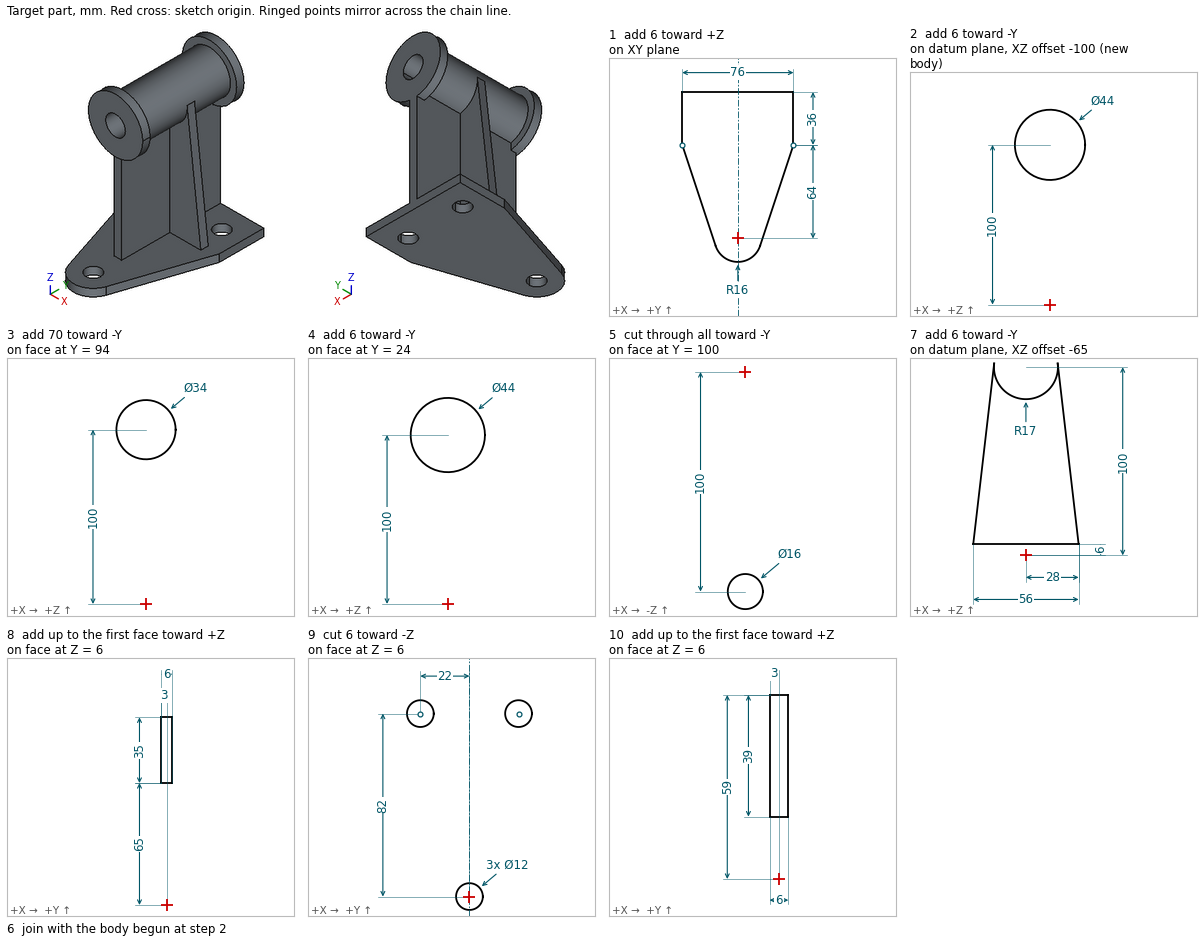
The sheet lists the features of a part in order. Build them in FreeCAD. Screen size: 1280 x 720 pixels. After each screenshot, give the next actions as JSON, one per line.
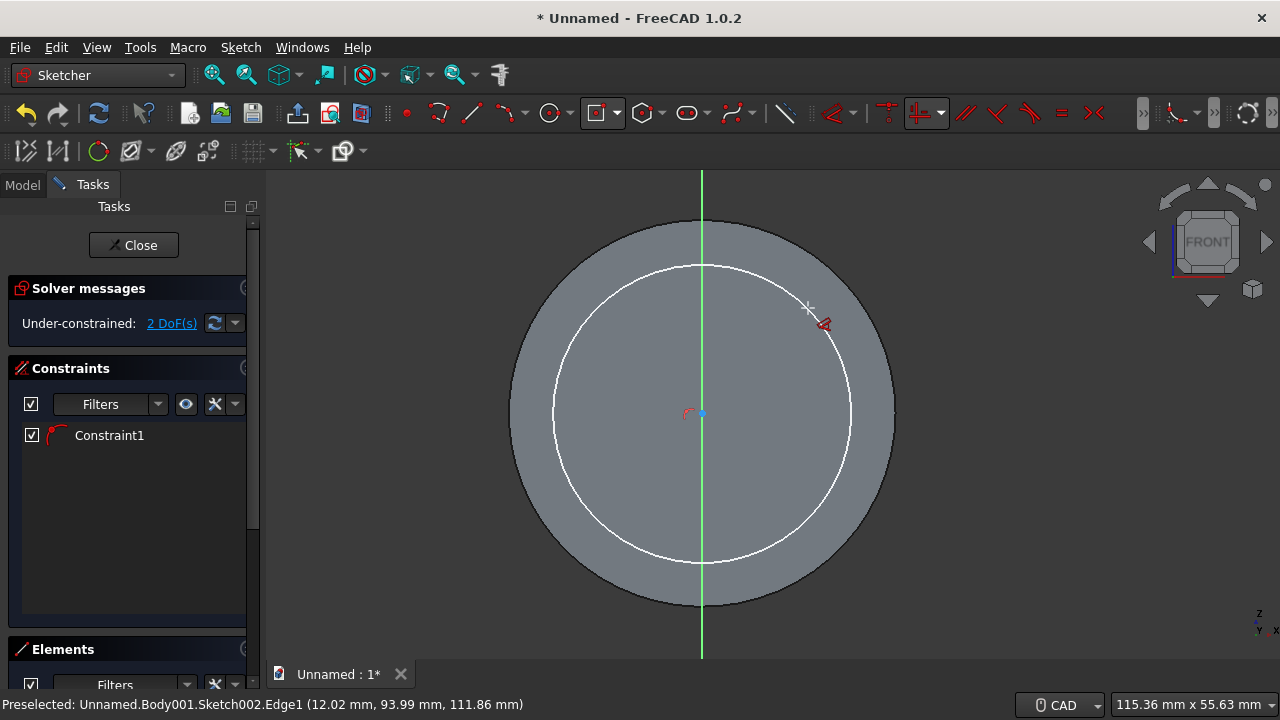
{"action": "left_click", "coordinate": [807, 308]}
{"action": "left_click", "coordinate": [830, 285]}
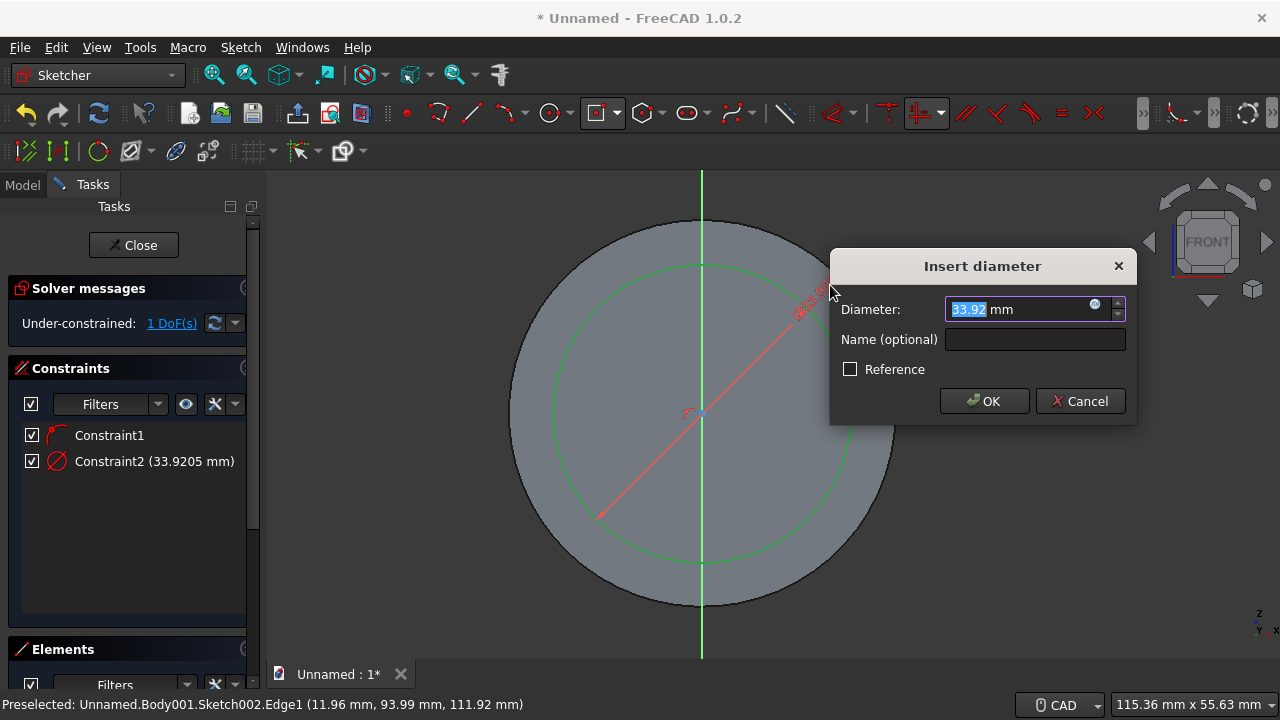
{"action": "type", "text": "34"}
{"action": "key", "text": "Return"}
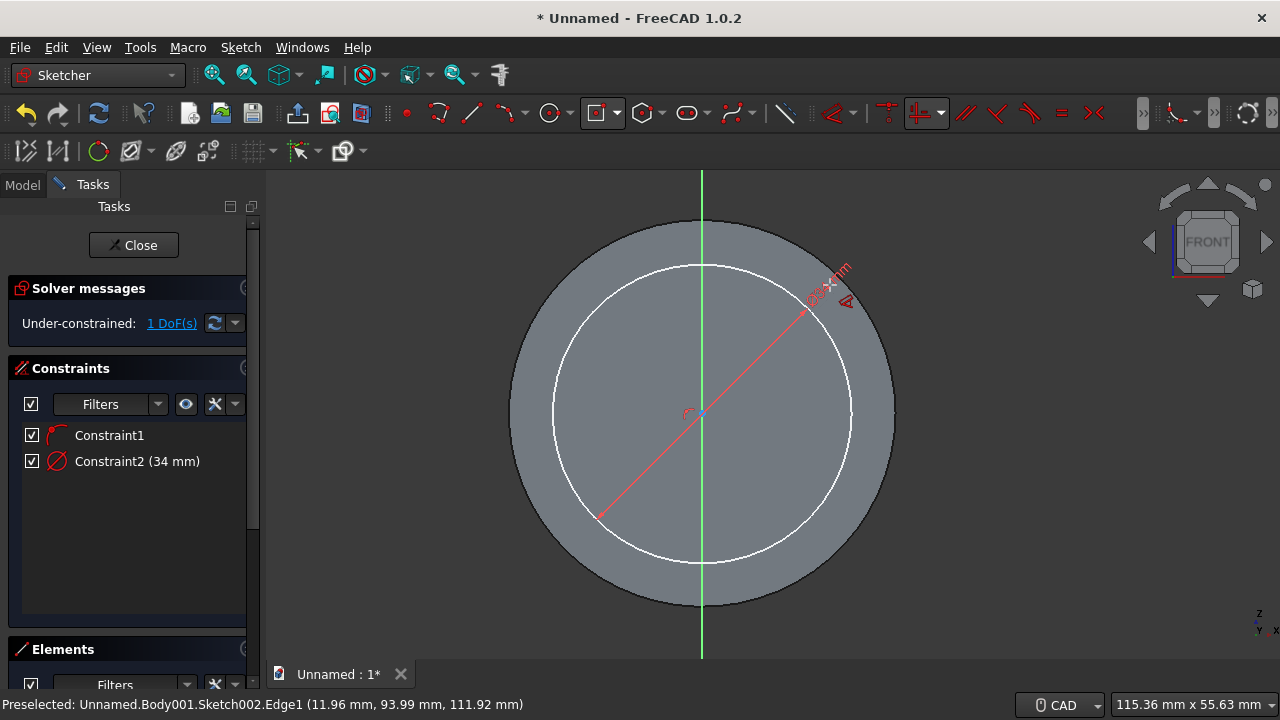
{"action": "left_click", "coordinate": [702, 414]}
{"action": "left_click", "coordinate": [736, 522]}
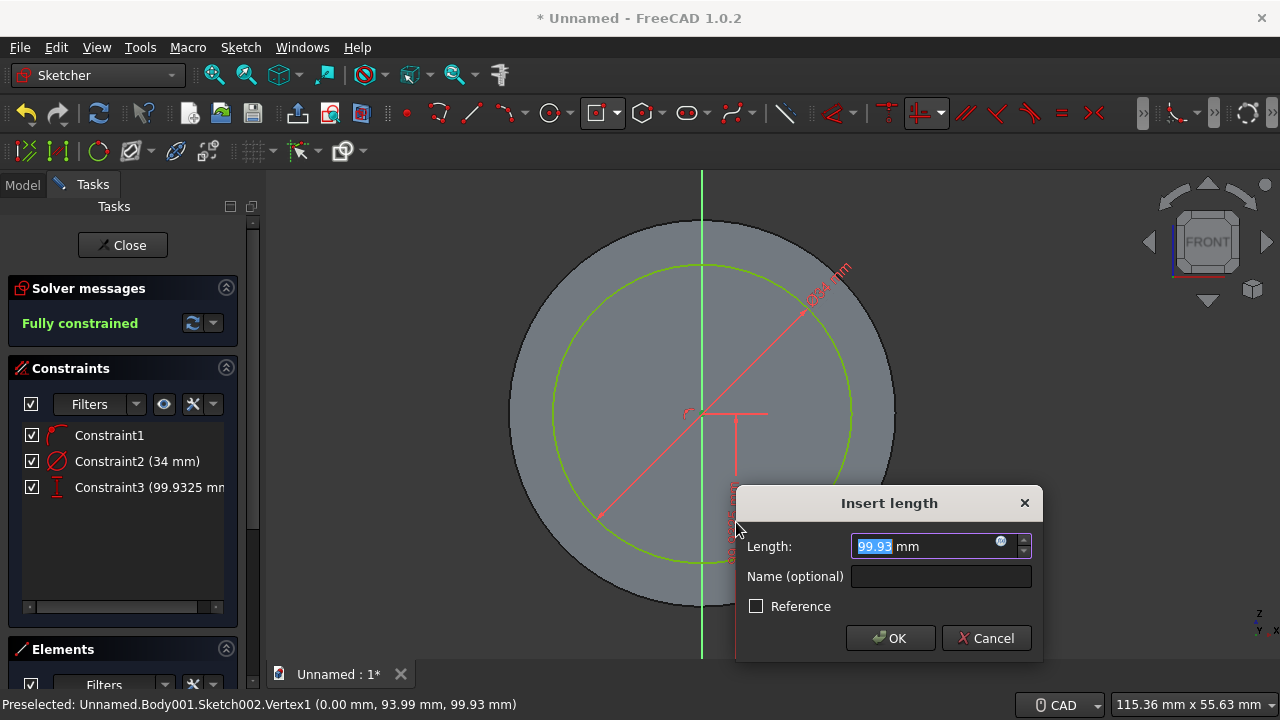
{"action": "type", "text": "100"}
{"action": "key", "text": "Return"}
{"action": "key", "text": "Escape"}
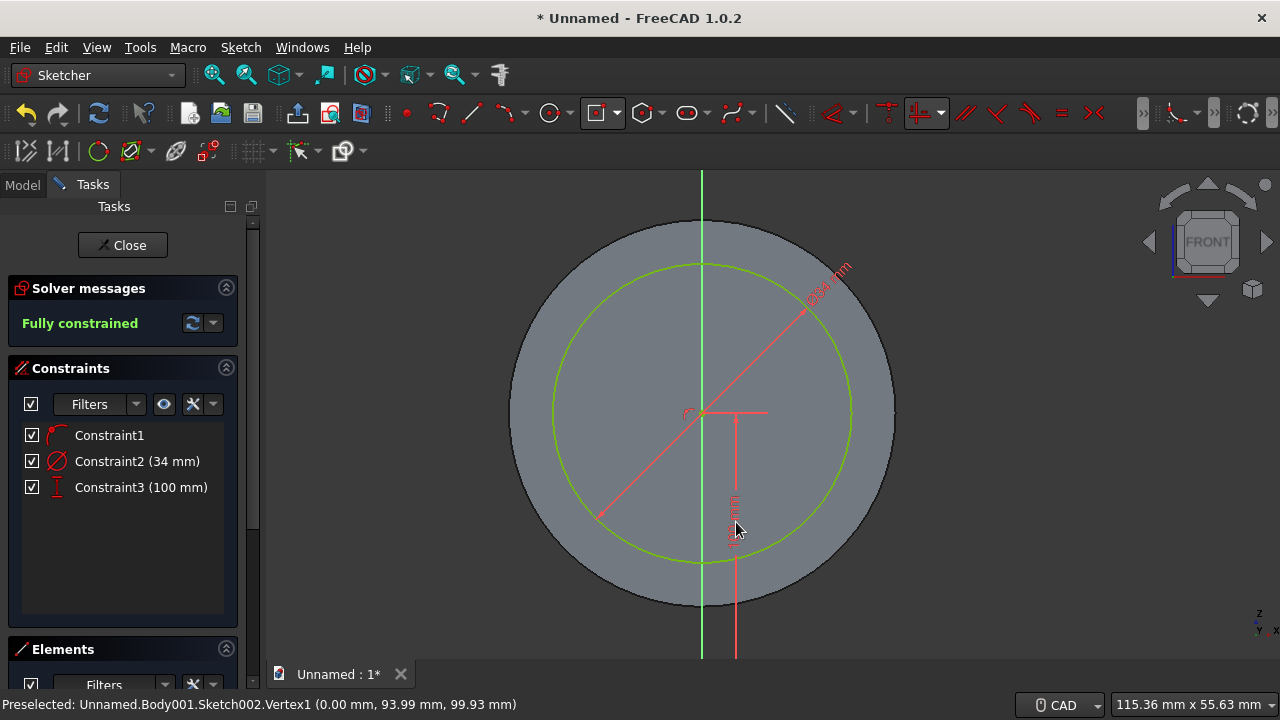
{"action": "left_click", "coordinate": [123, 245]}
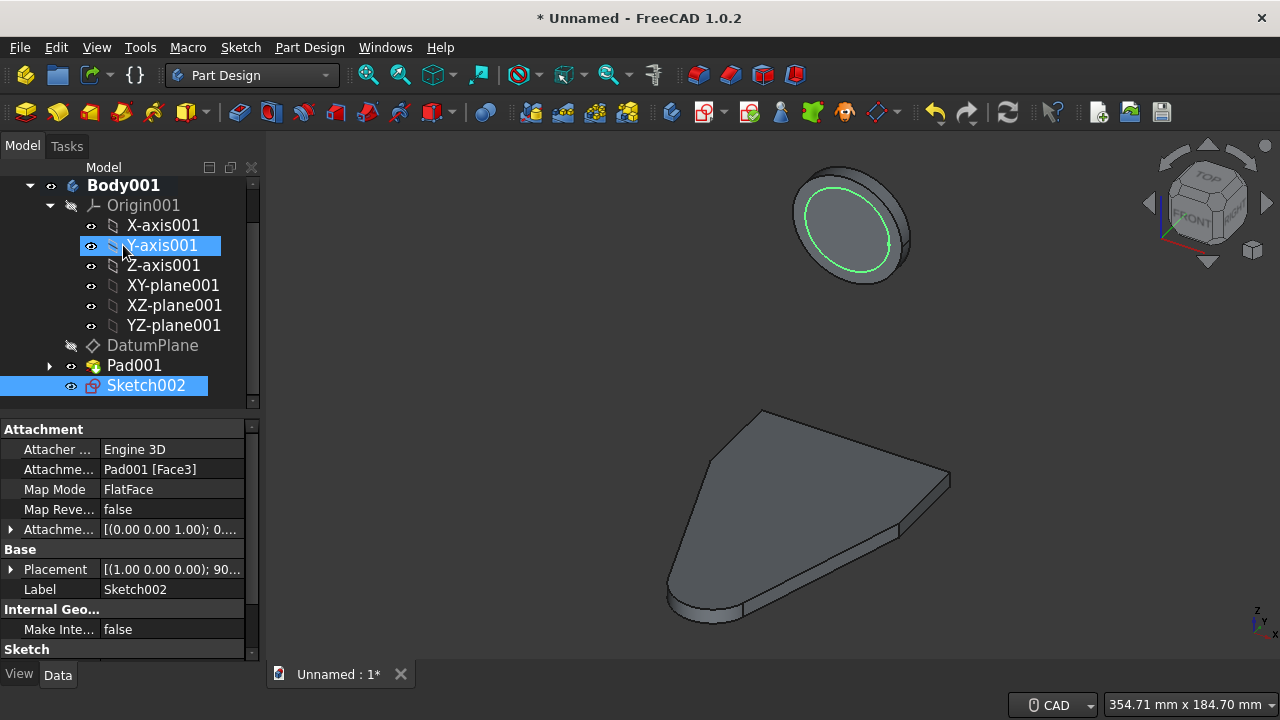
{"action": "left_click", "coordinate": [26, 112]}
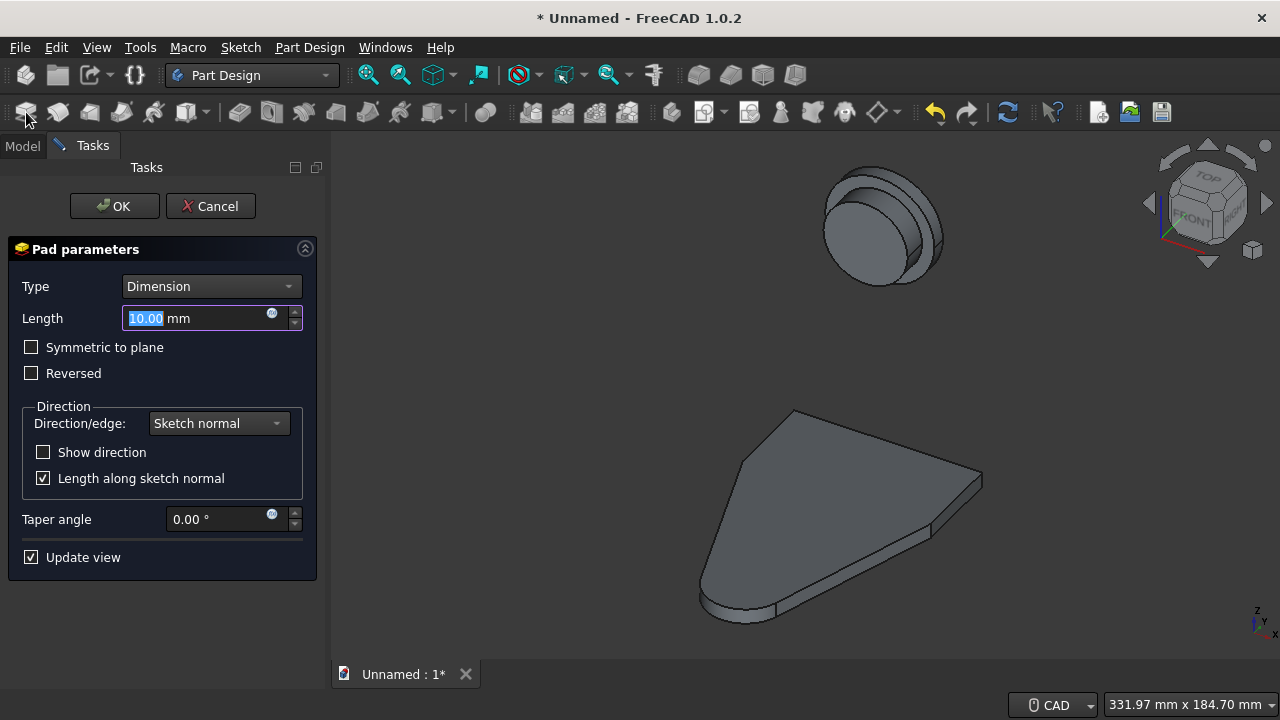
{"action": "type", "text": "70"}
{"action": "key", "text": "Tab"}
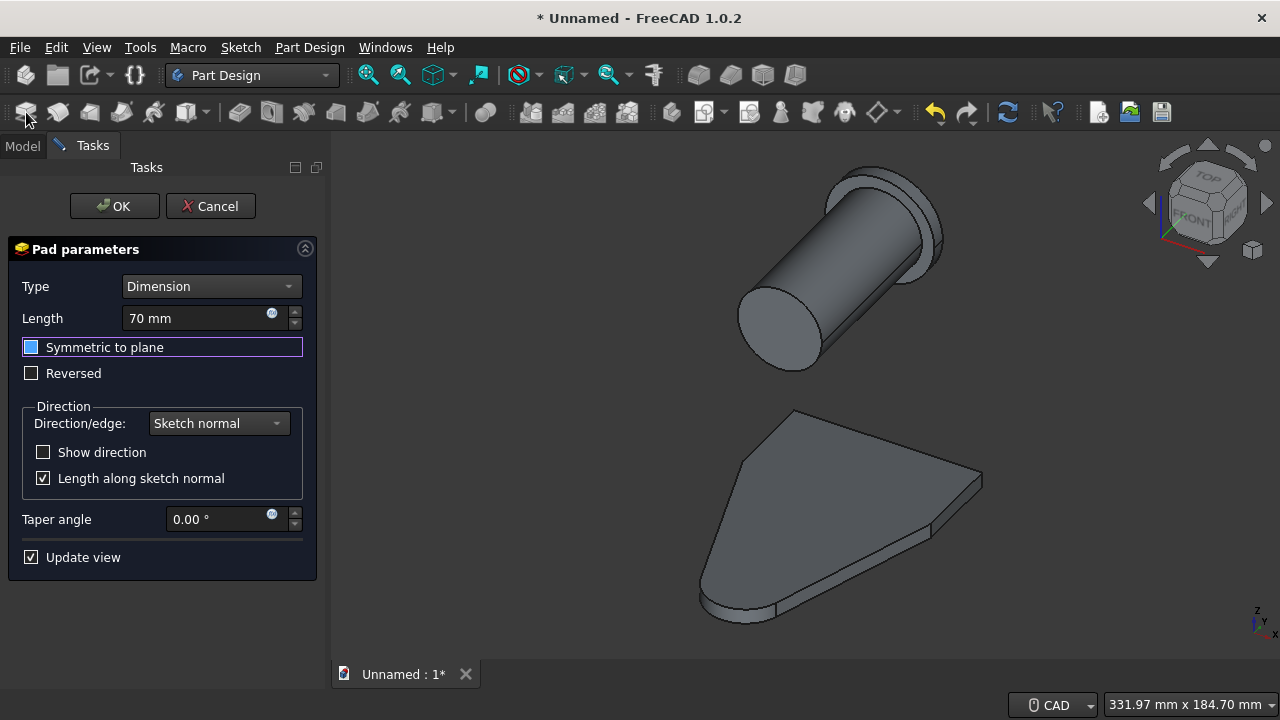
{"action": "left_click", "coordinate": [115, 206]}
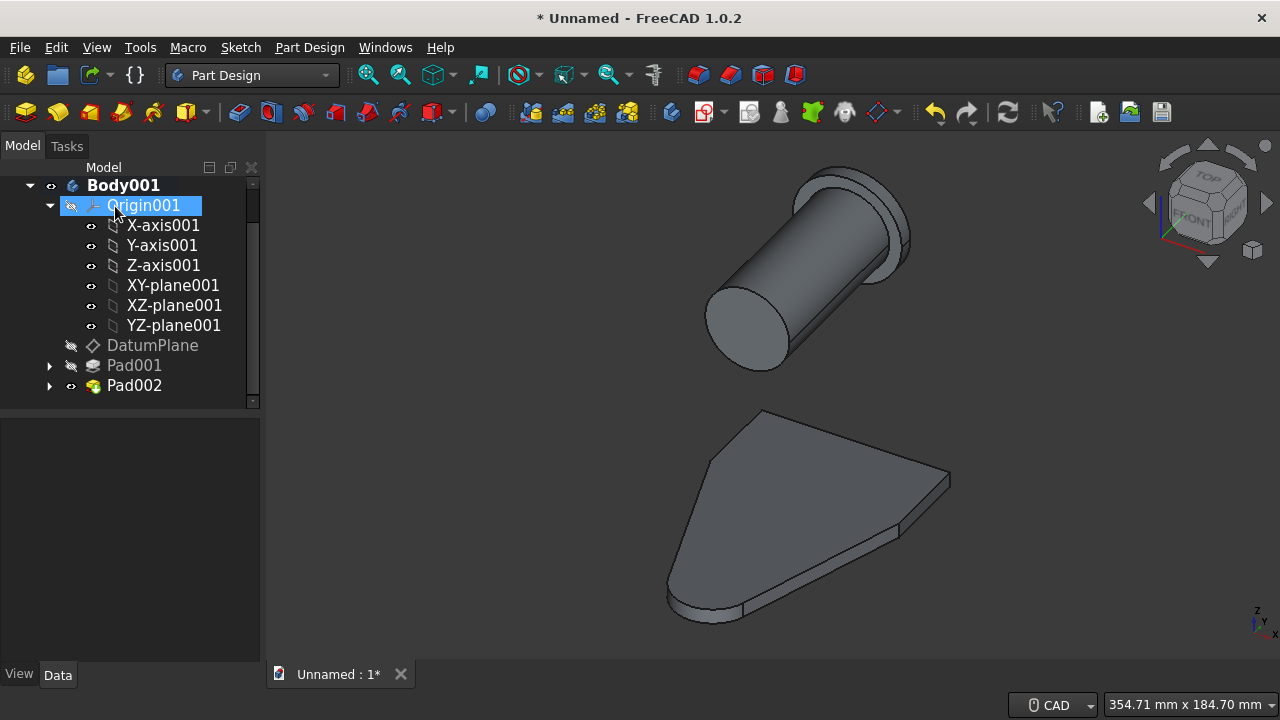
{"action": "left_click", "coordinate": [747, 328]}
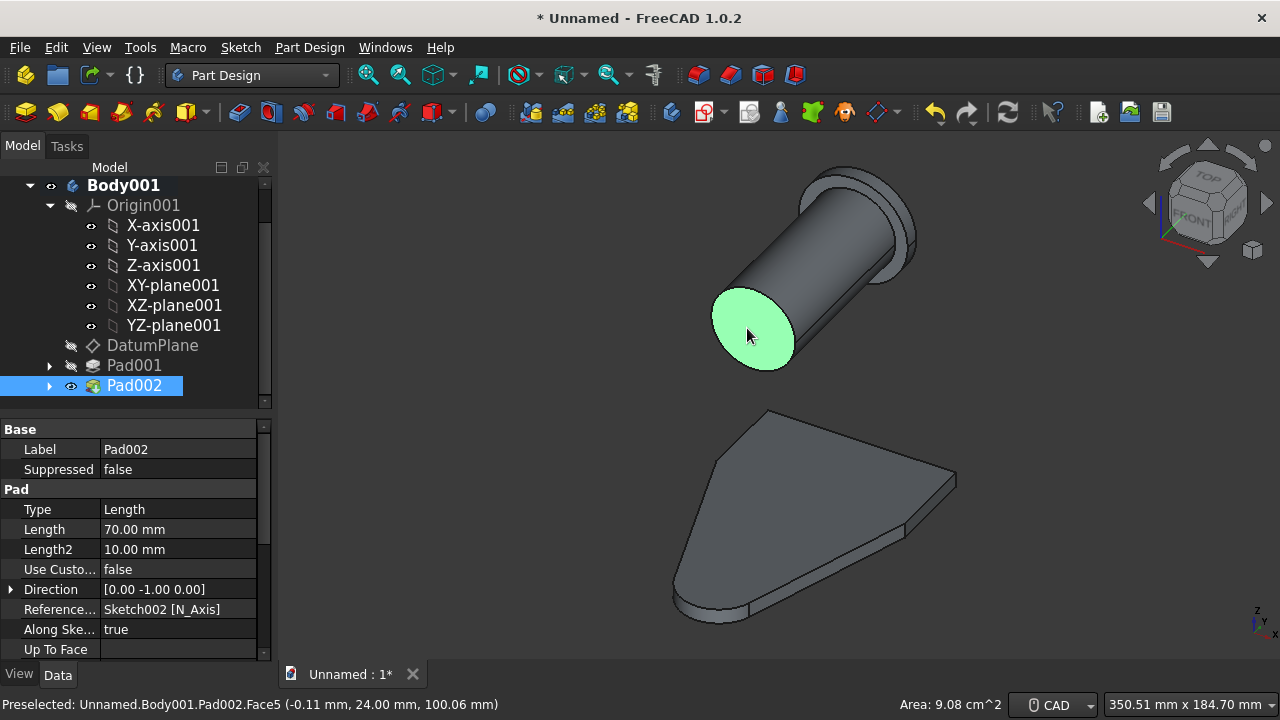
{"action": "left_click", "coordinate": [704, 112]}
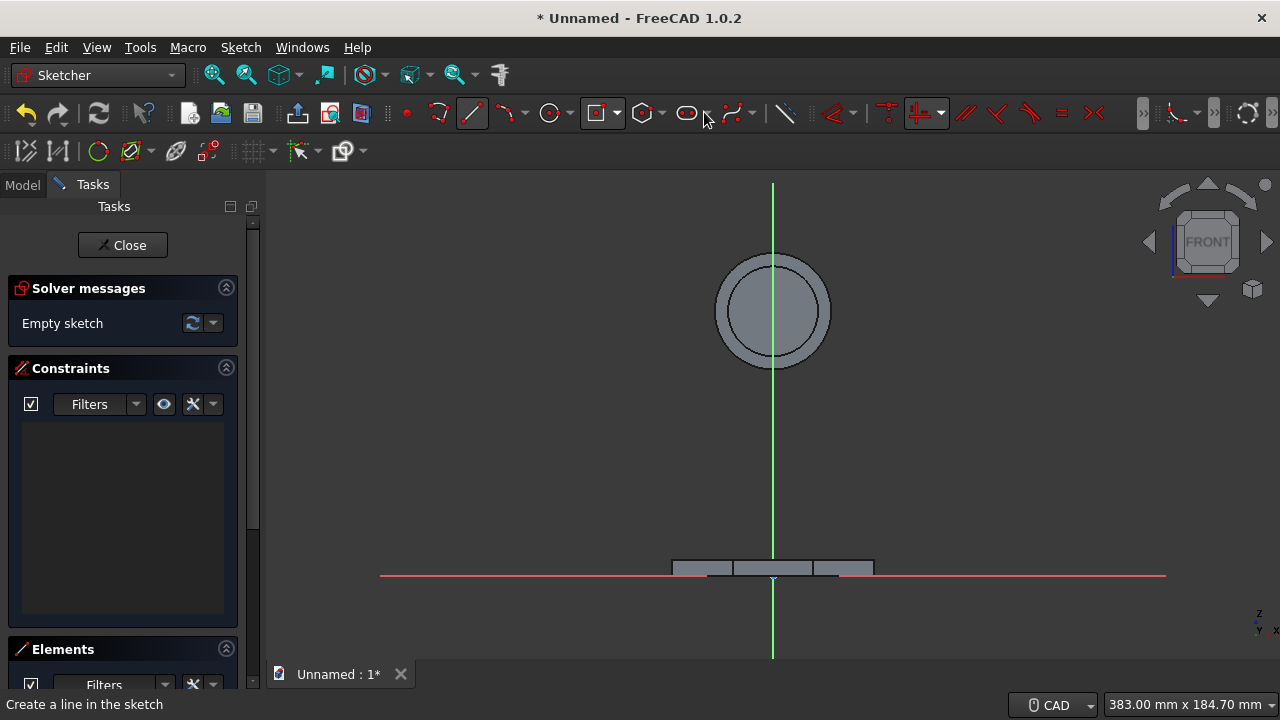
{"action": "scroll", "coordinate": [813, 251], "scroll_direction": "up", "scroll_amount": 5}